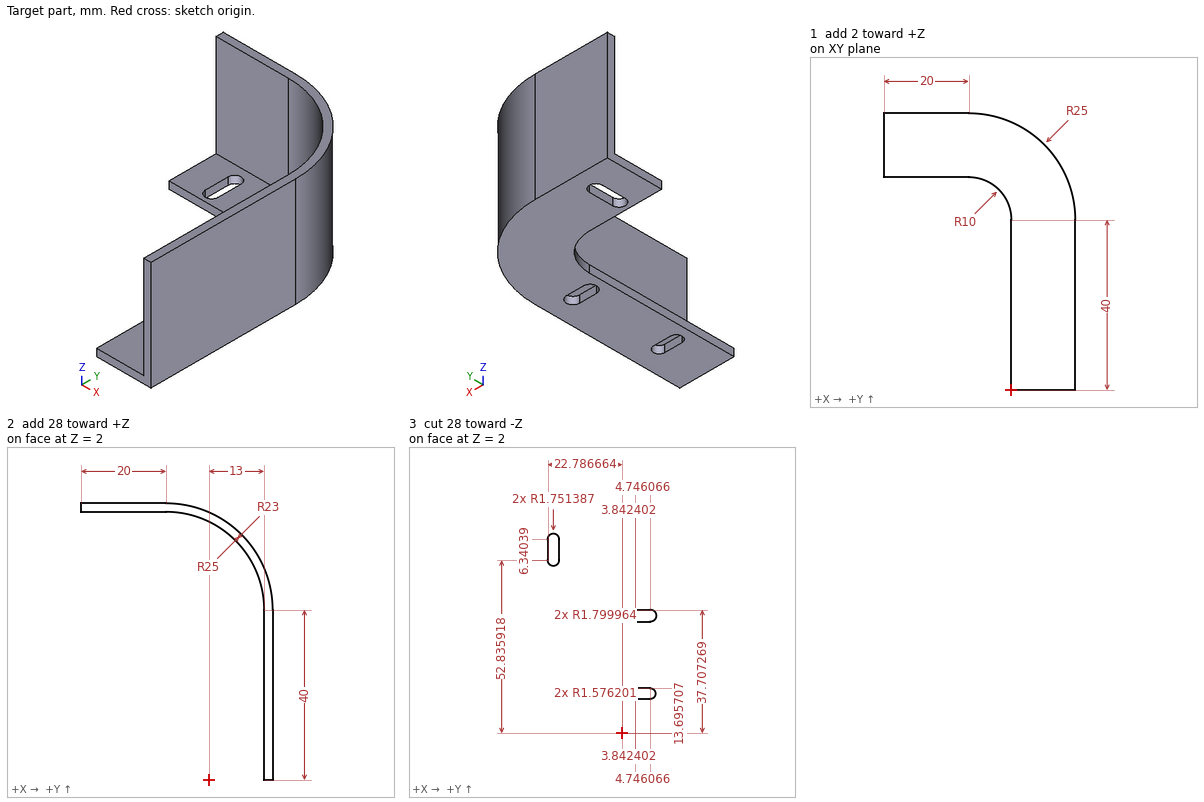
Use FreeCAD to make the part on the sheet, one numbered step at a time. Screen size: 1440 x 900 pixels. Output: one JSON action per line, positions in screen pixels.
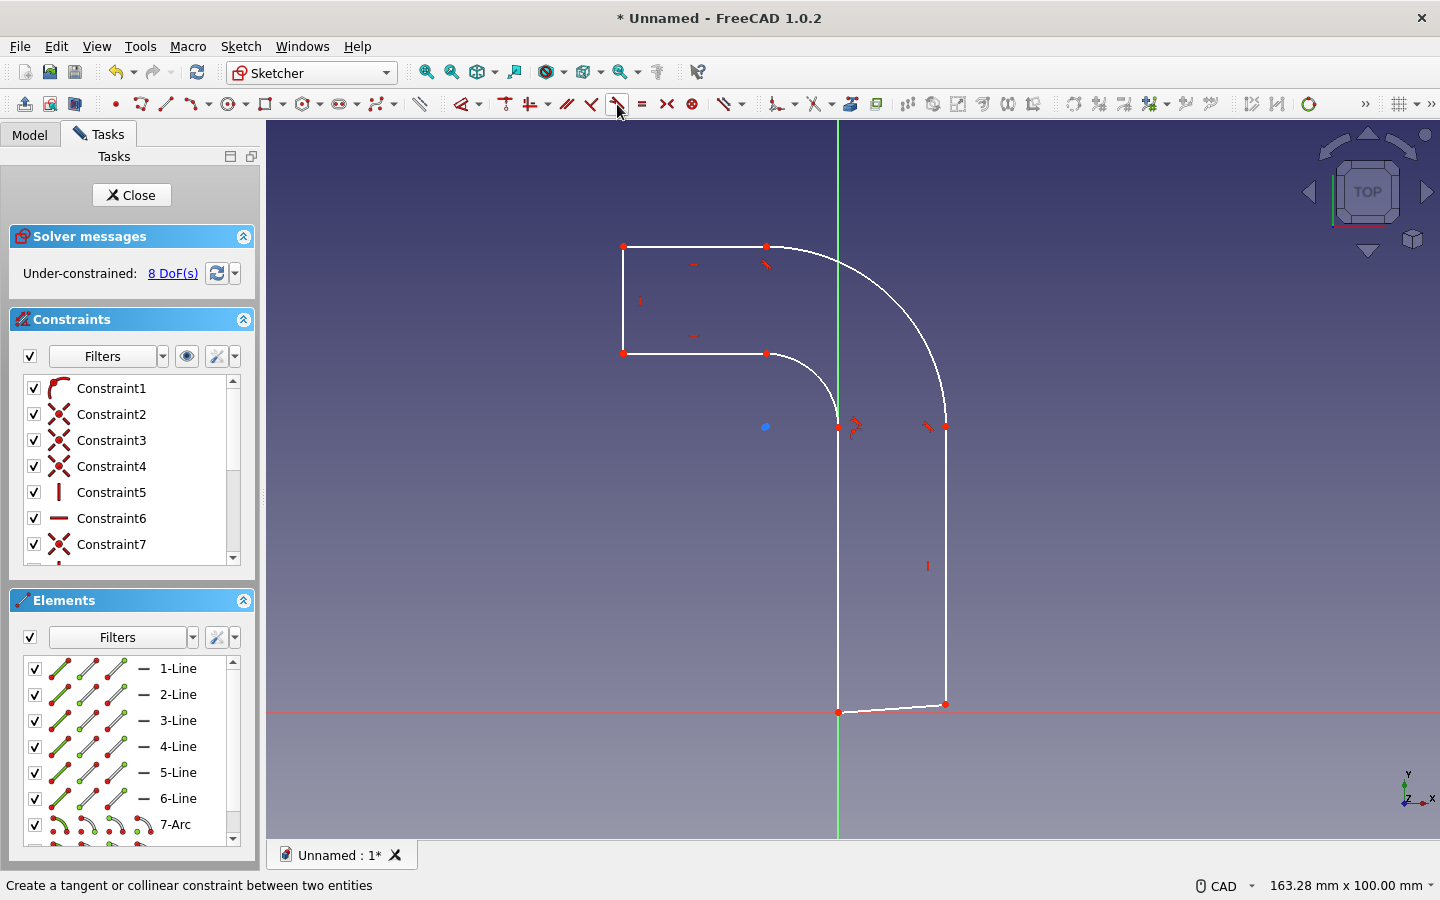
{"action": "left_click", "coordinate": [666, 354]}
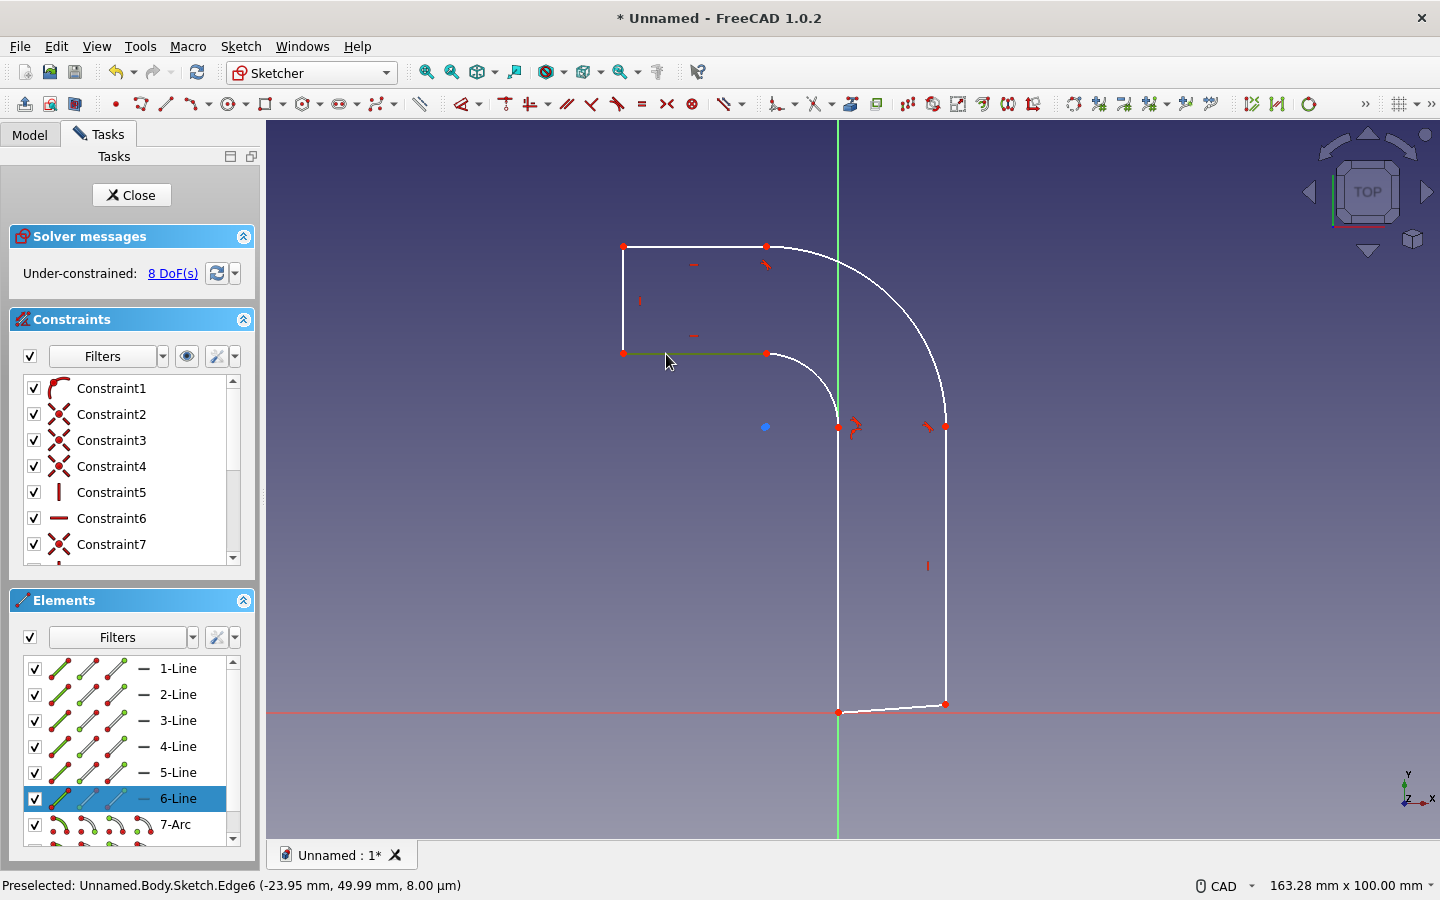
{"action": "left_click", "coordinate": [799, 362]}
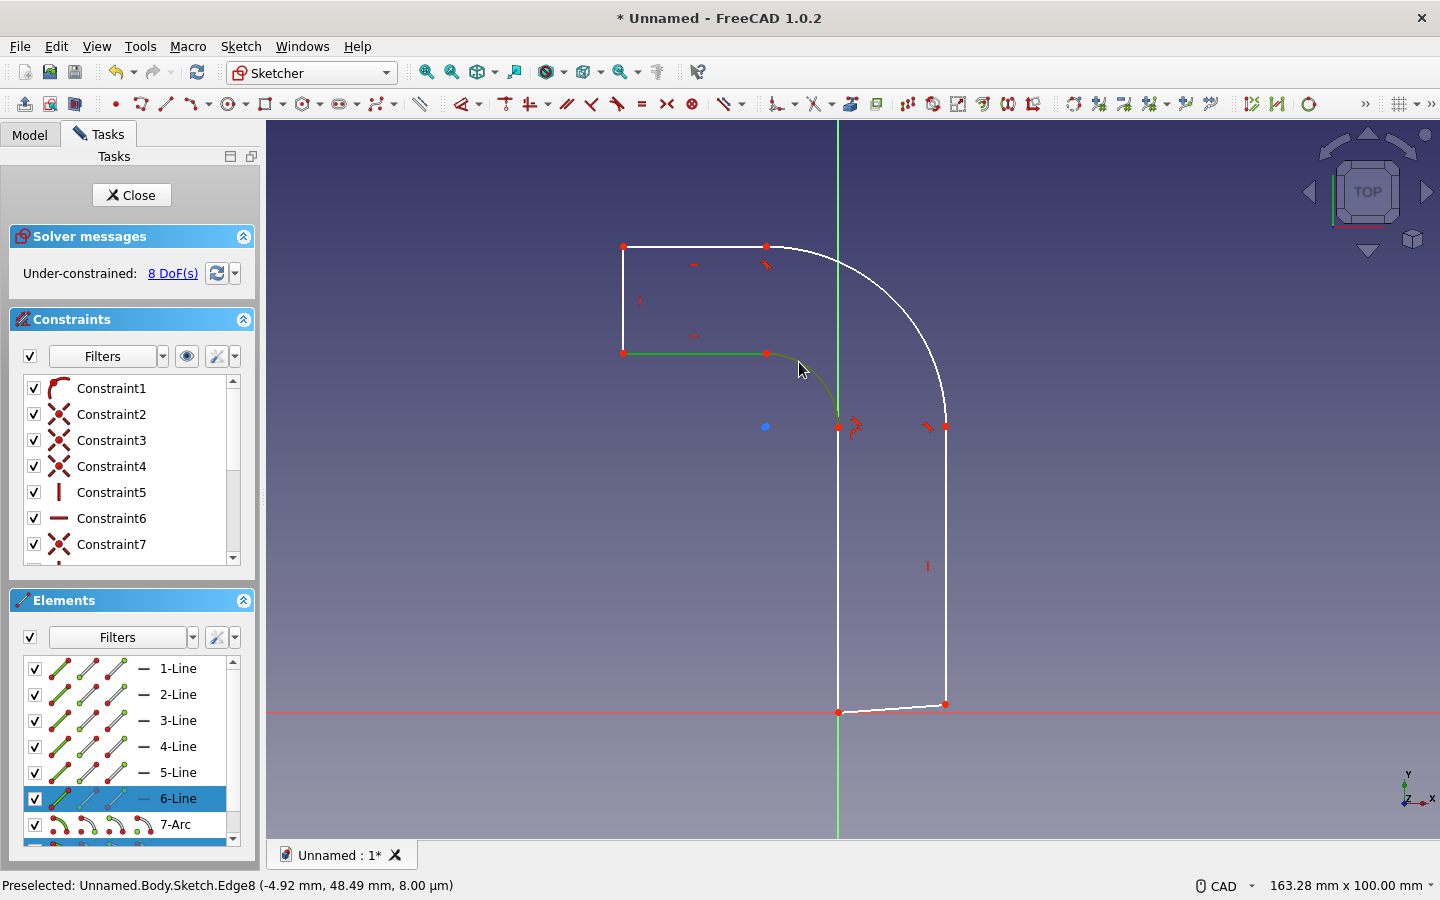
{"action": "left_click", "coordinate": [617, 104]}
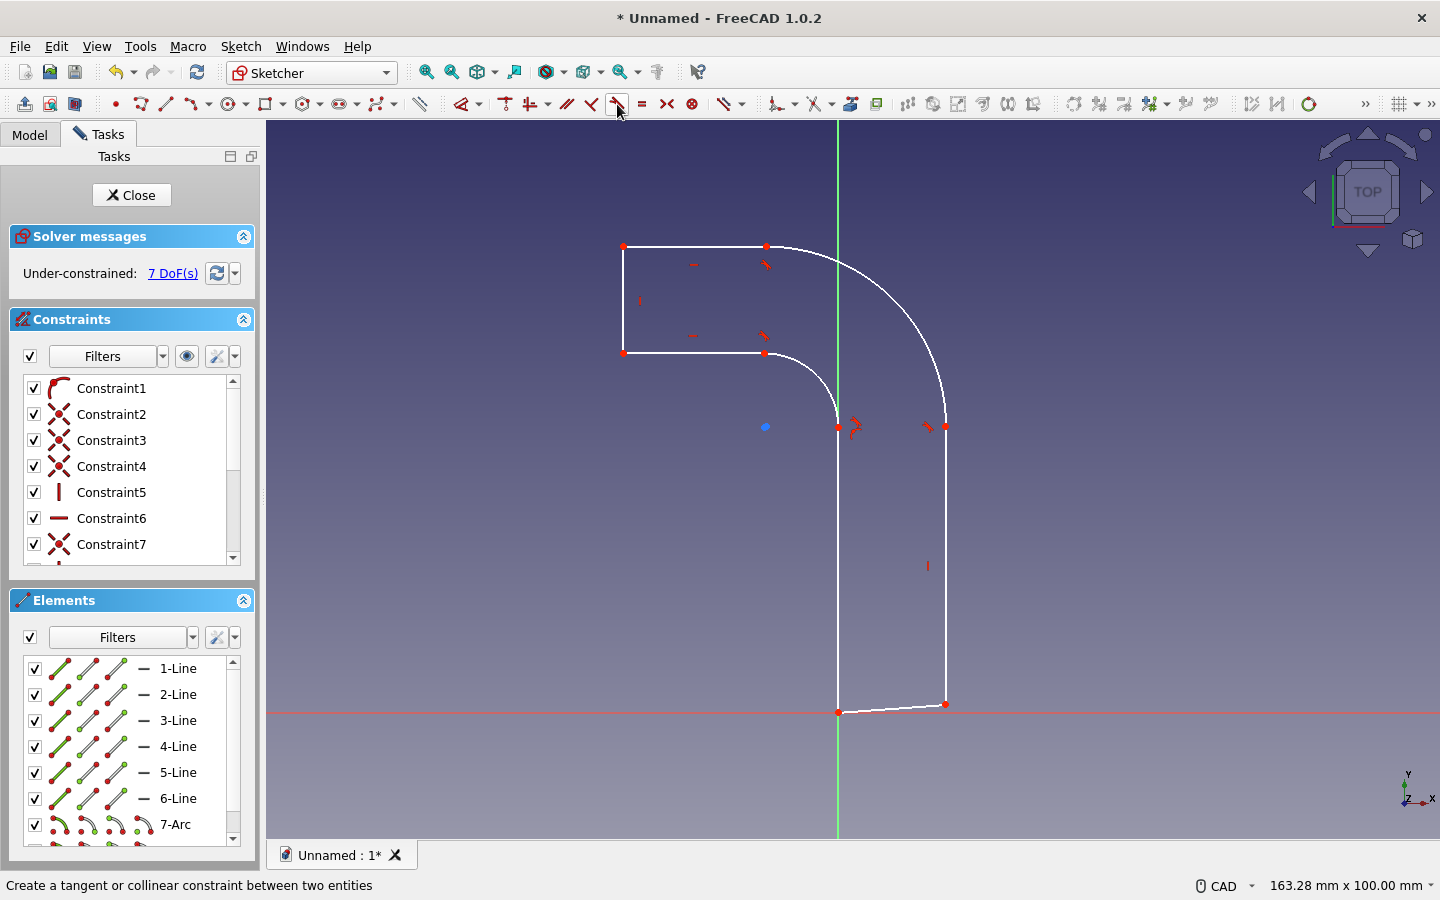
{"action": "left_click", "coordinate": [871, 711]}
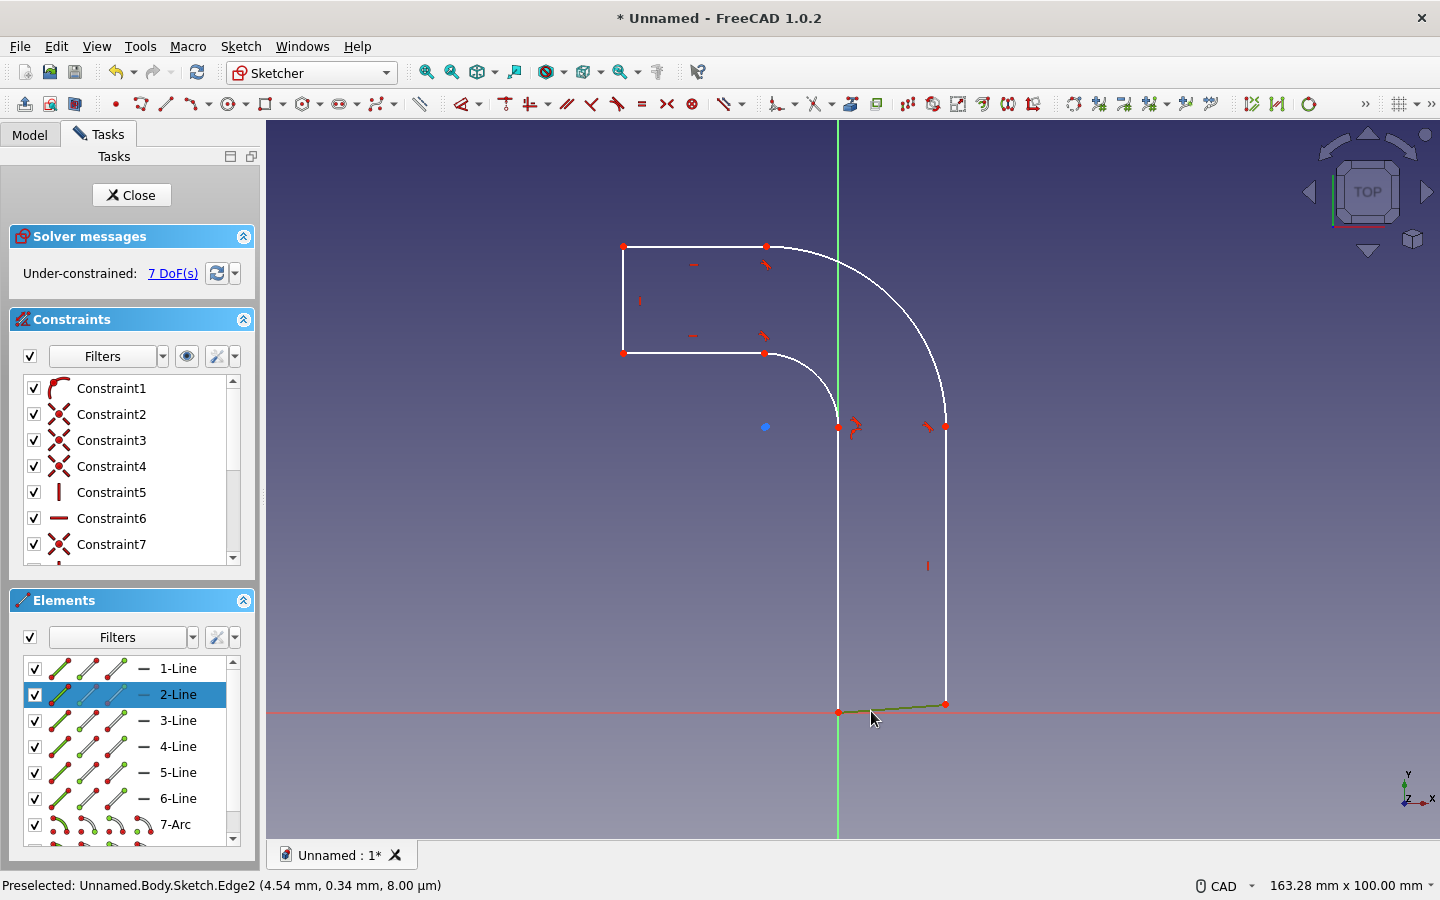
{"action": "left_click", "coordinate": [548, 104]}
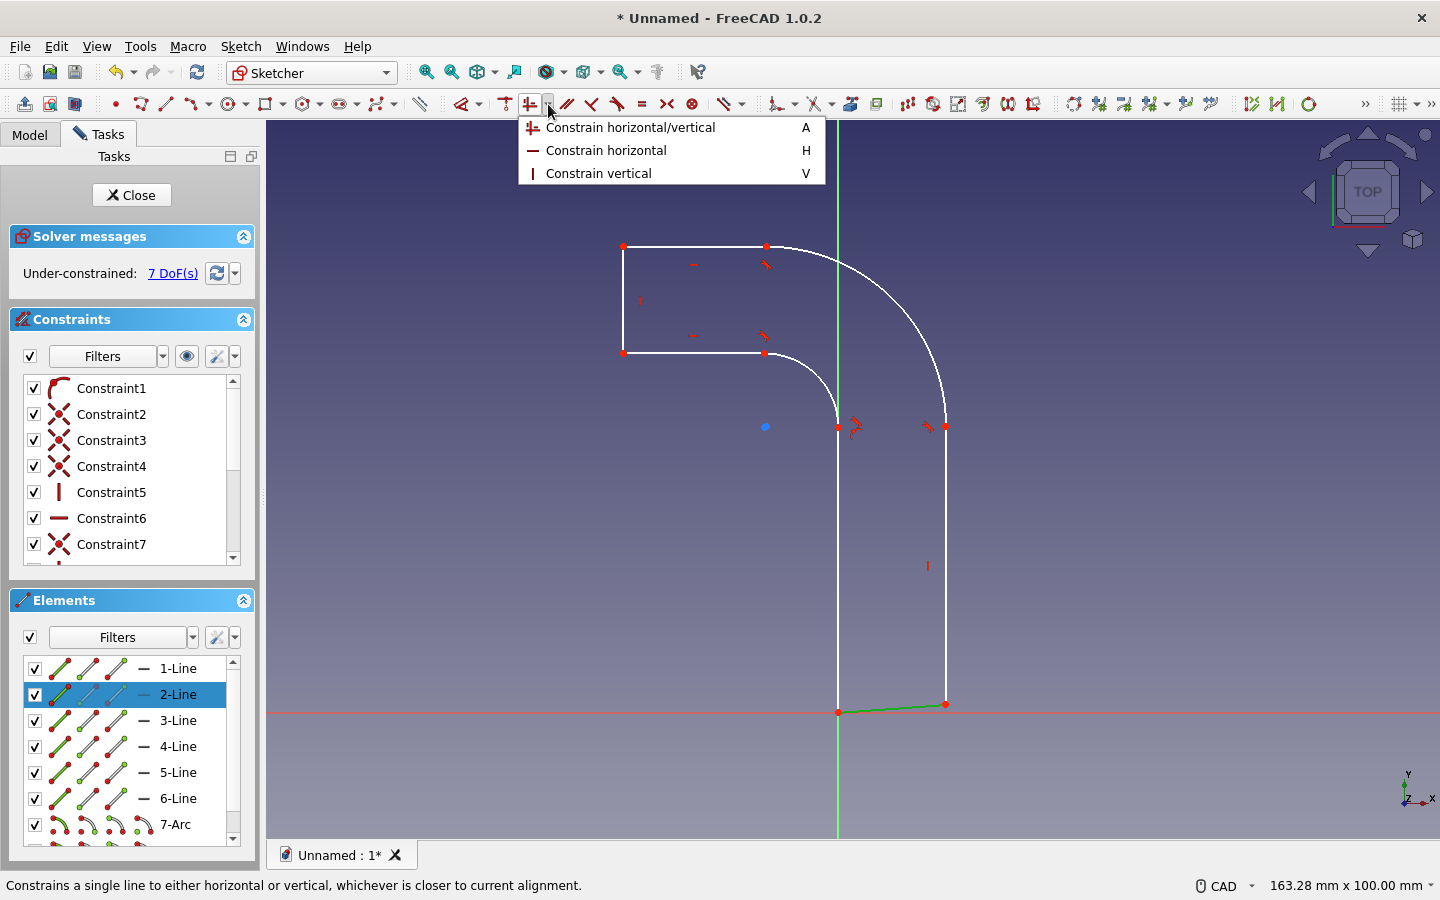
{"action": "left_click", "coordinate": [672, 150]}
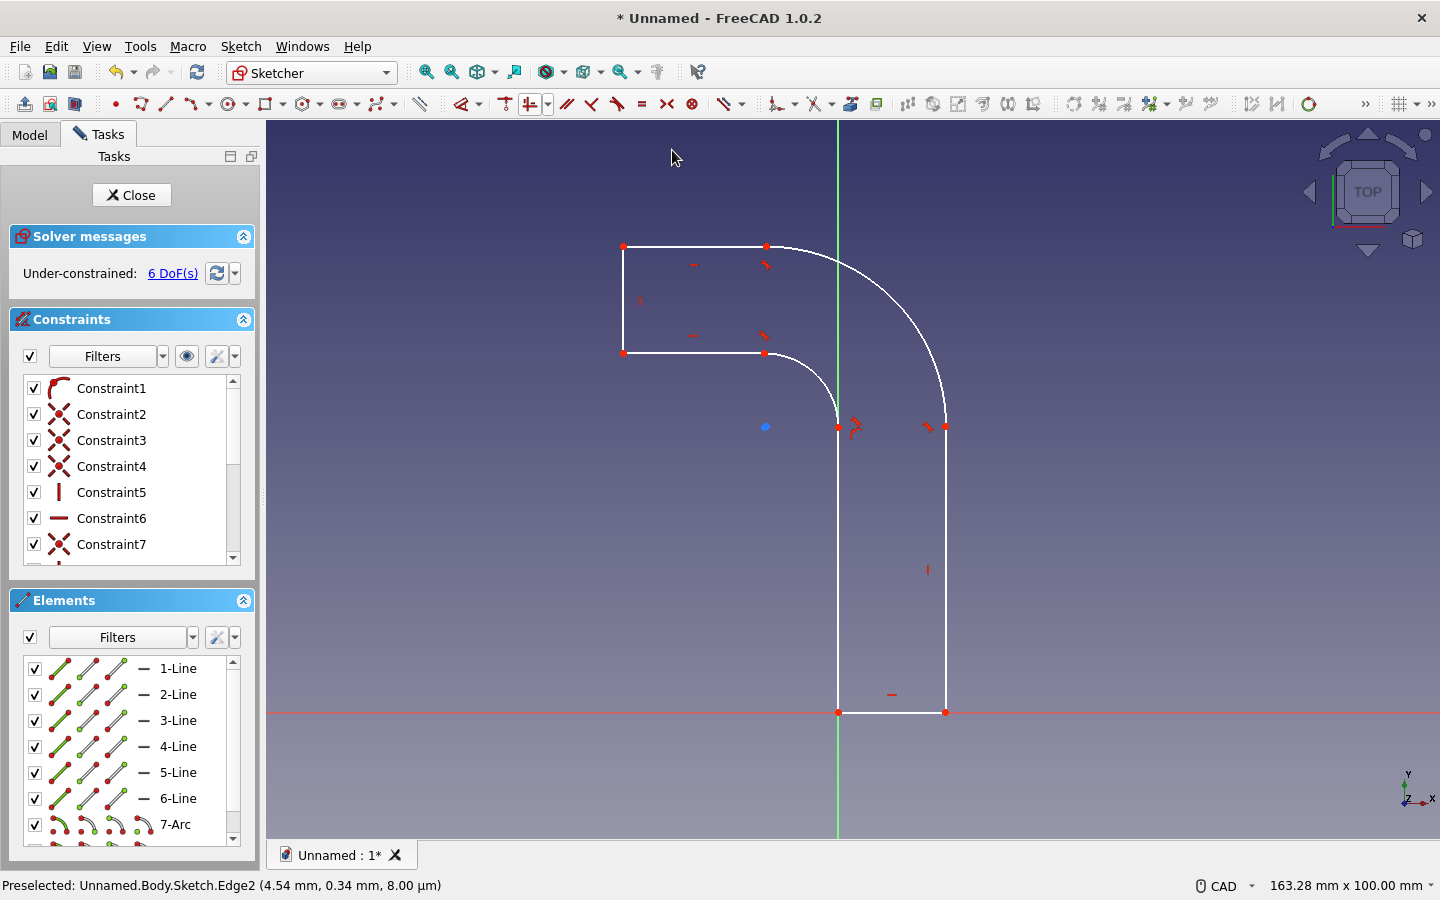
{"action": "left_click", "coordinate": [926, 345]}